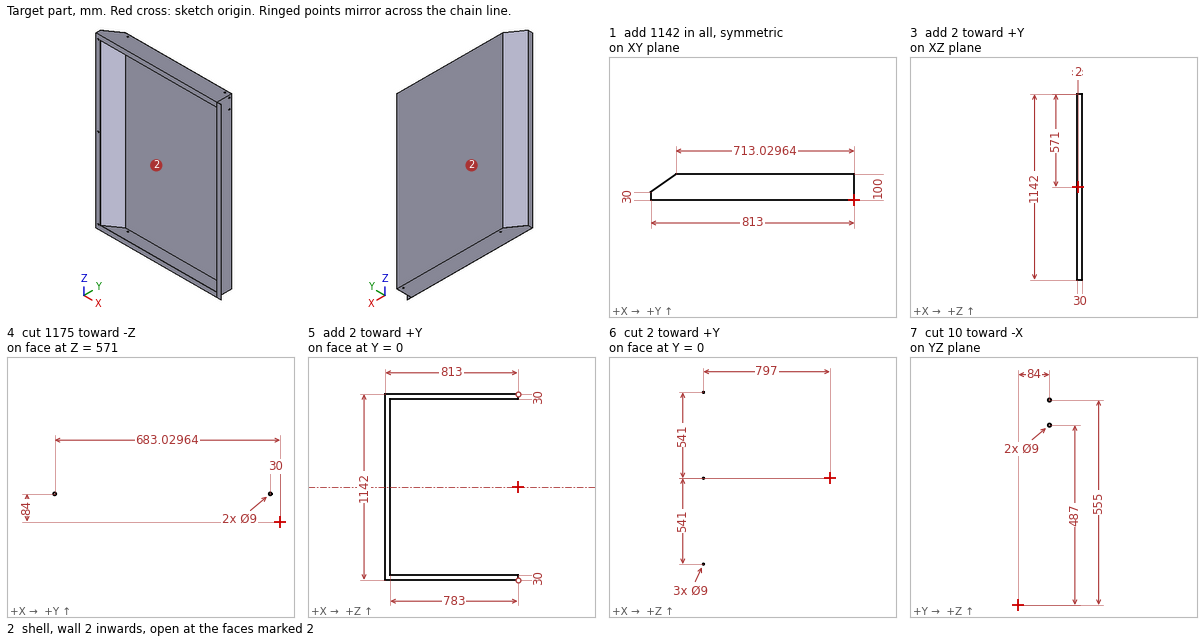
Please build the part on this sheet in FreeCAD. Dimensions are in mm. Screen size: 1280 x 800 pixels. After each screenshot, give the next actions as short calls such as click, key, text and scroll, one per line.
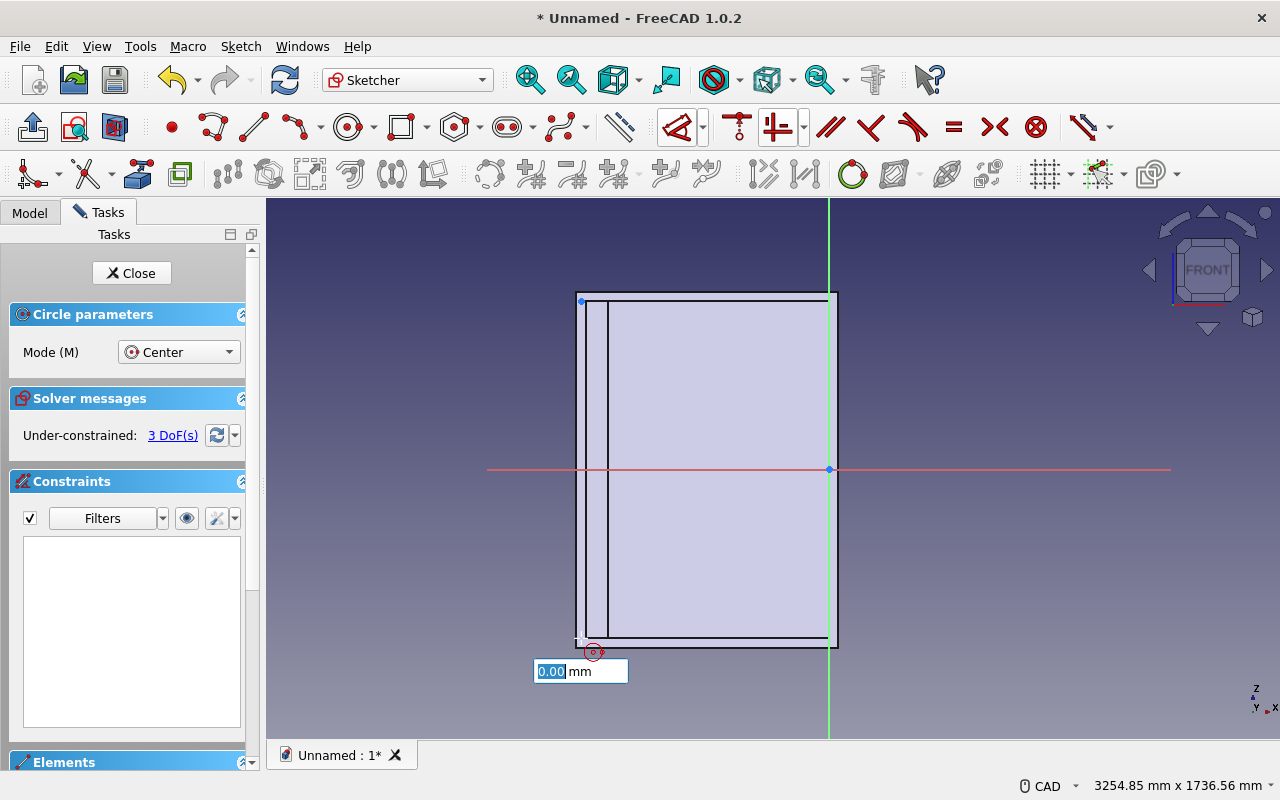
scroll(582, 637, up, 13)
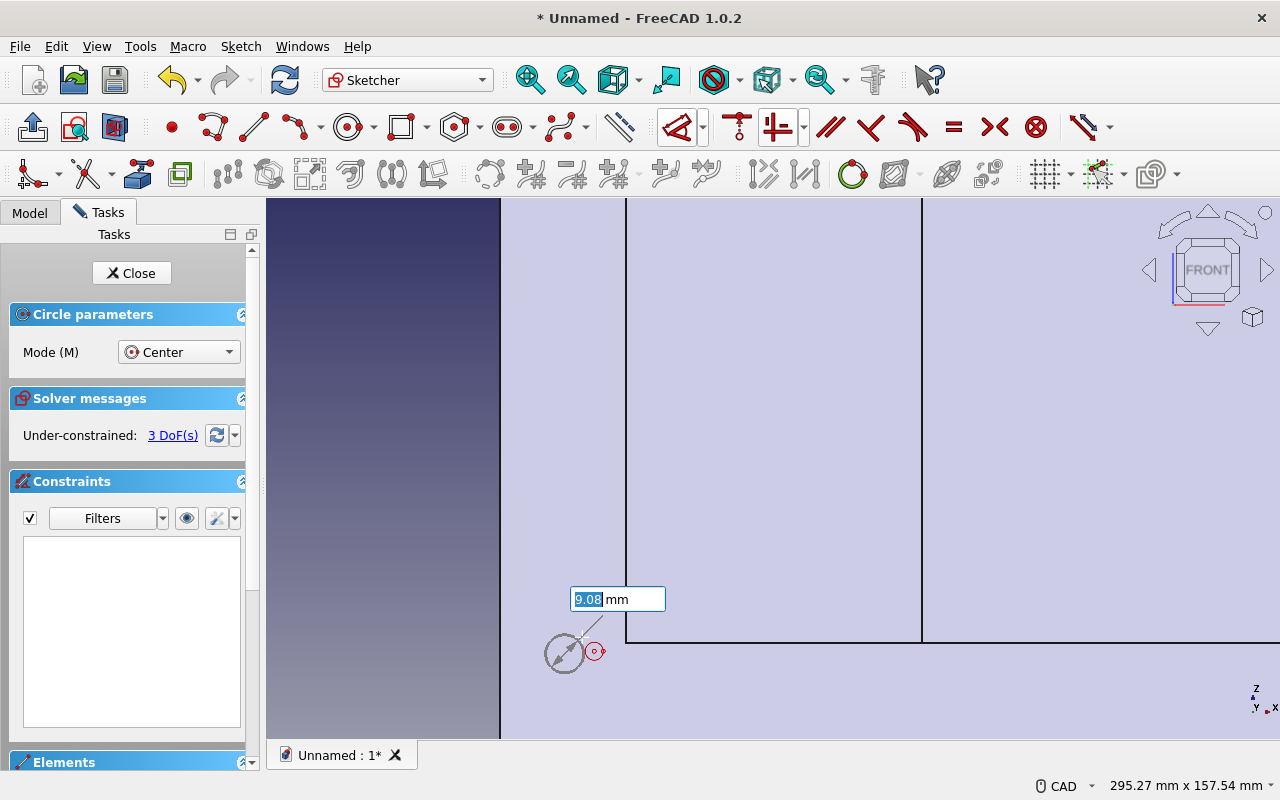
click(580, 629)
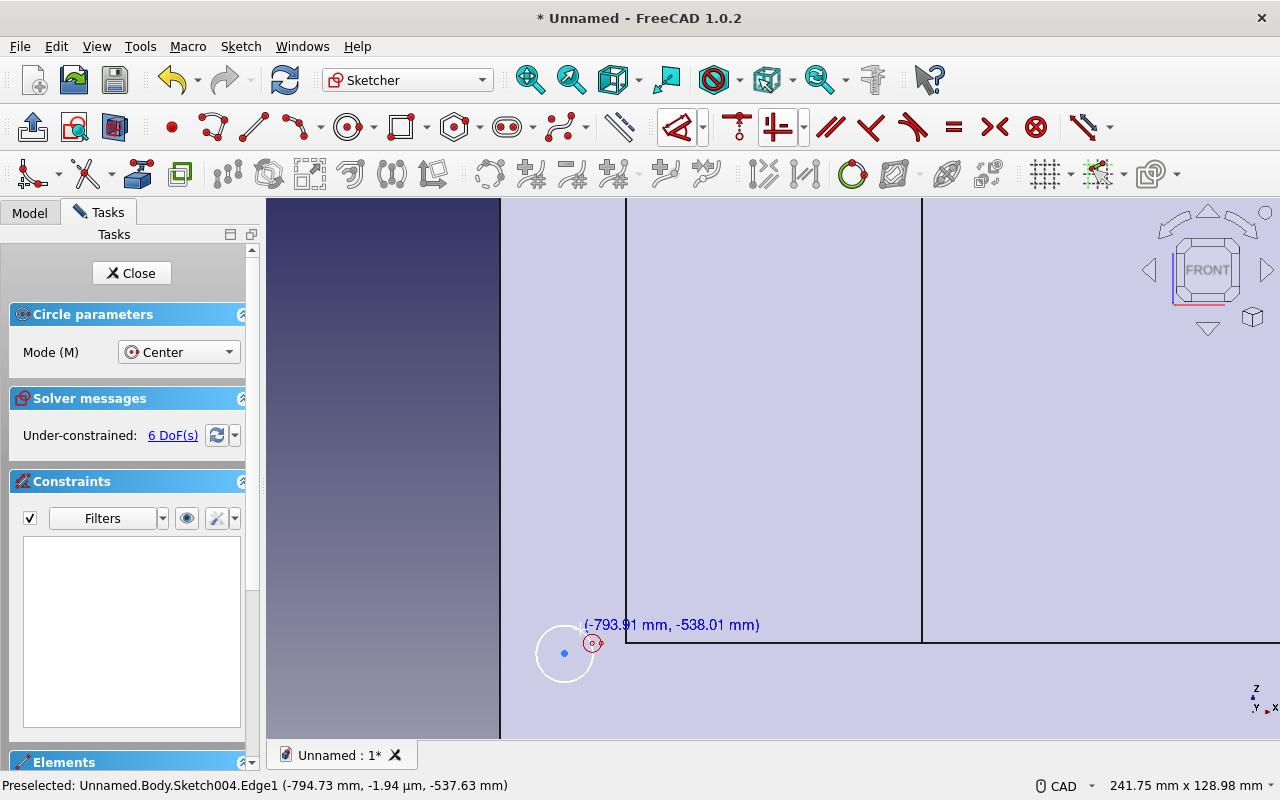
scroll(582, 637, down, 13)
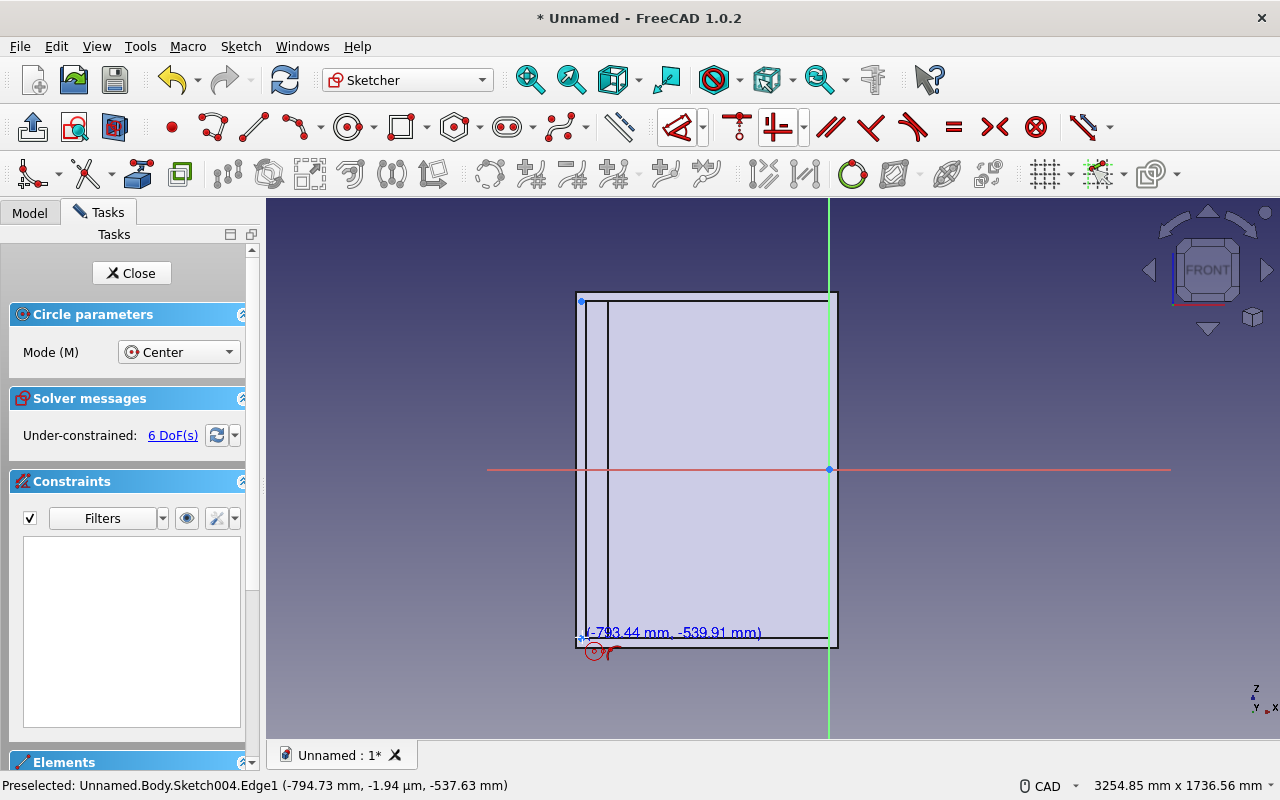
scroll(581, 470, up, 14)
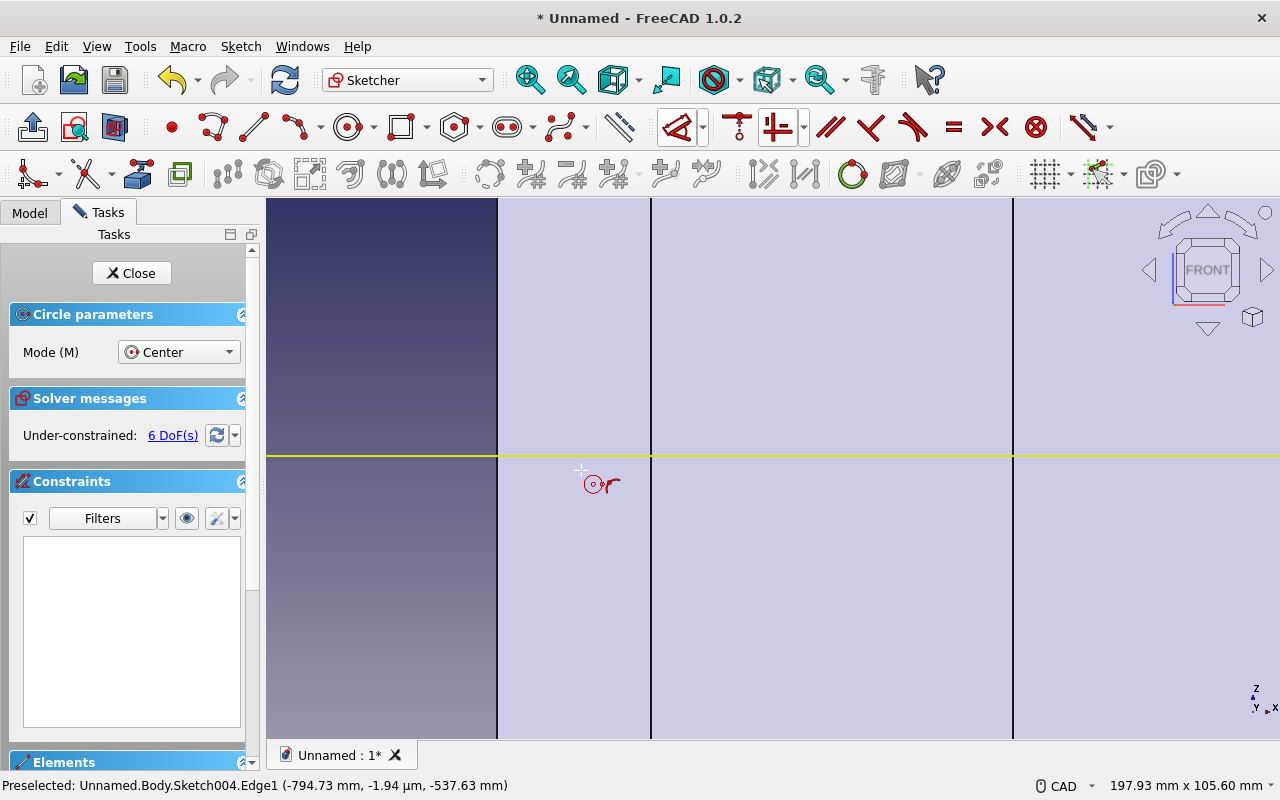
scroll(581, 469, down, 14)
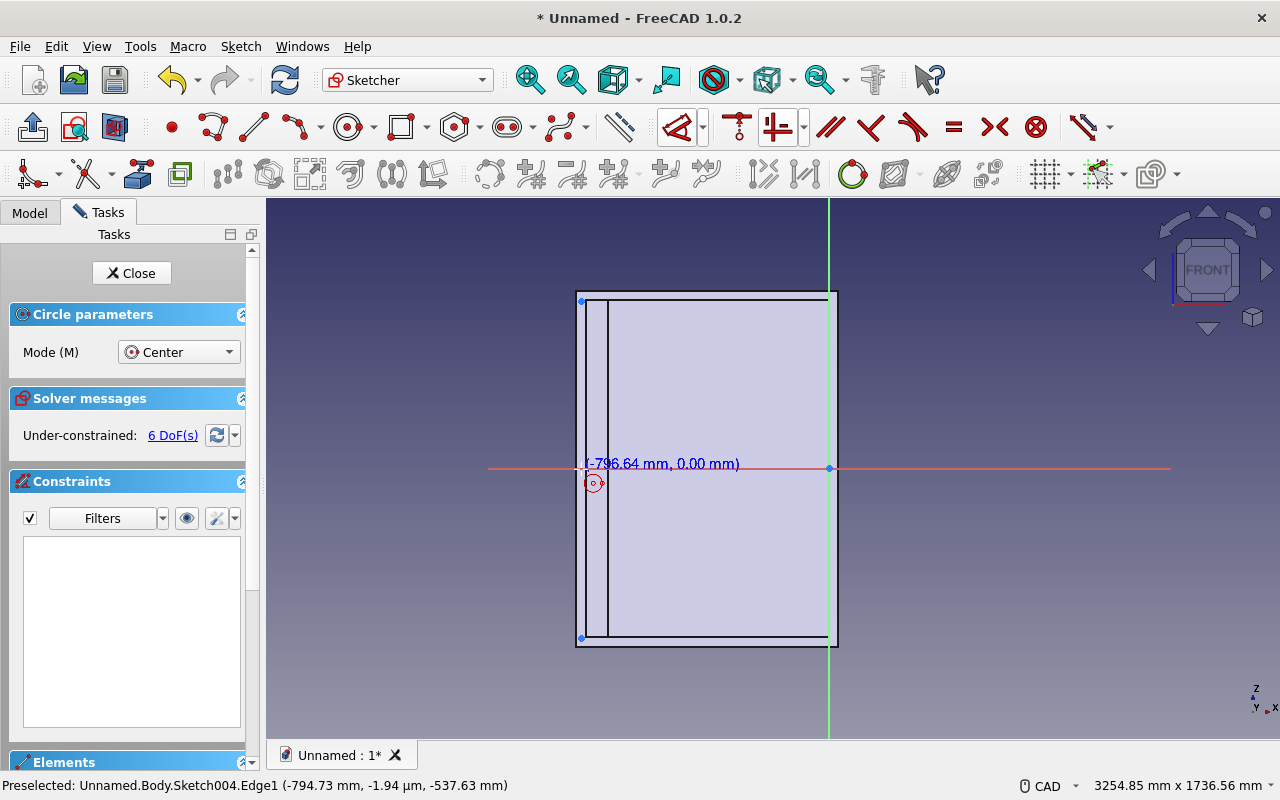
click(581, 469)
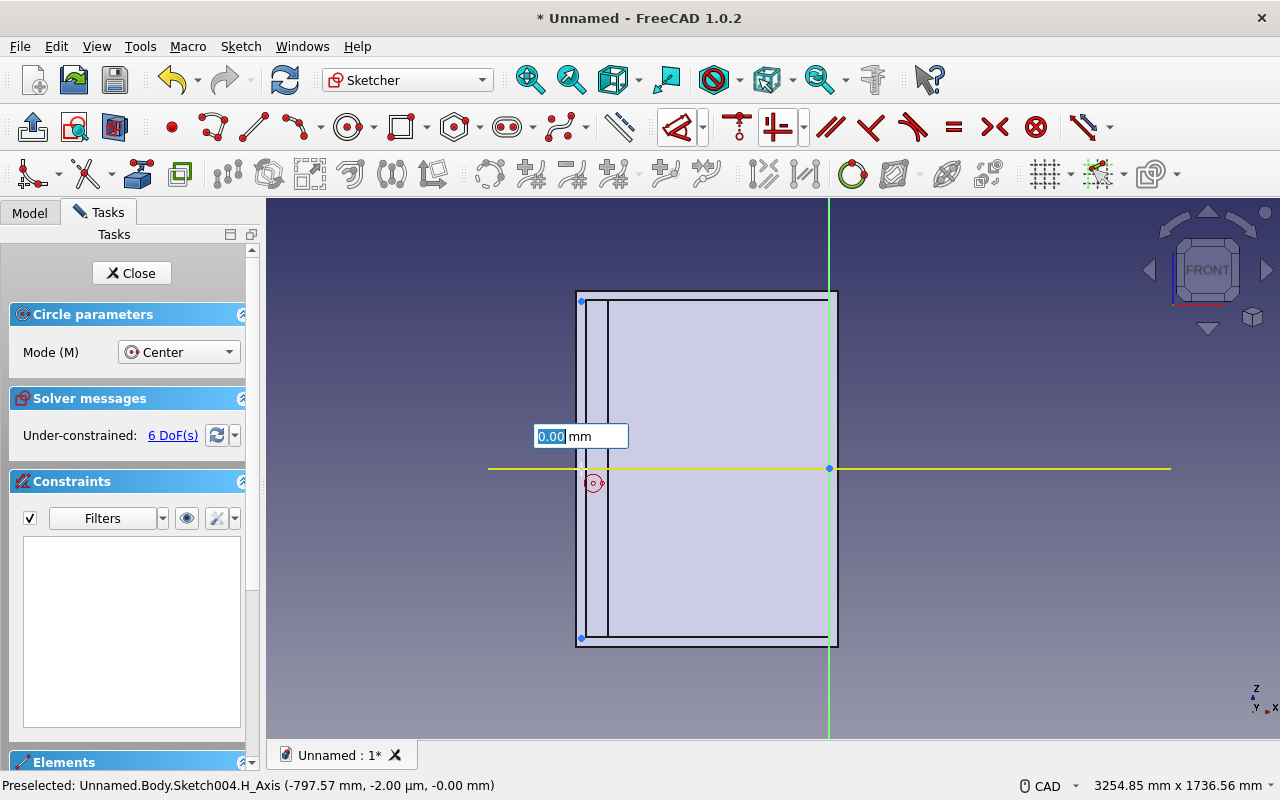
scroll(581, 470, up, 13)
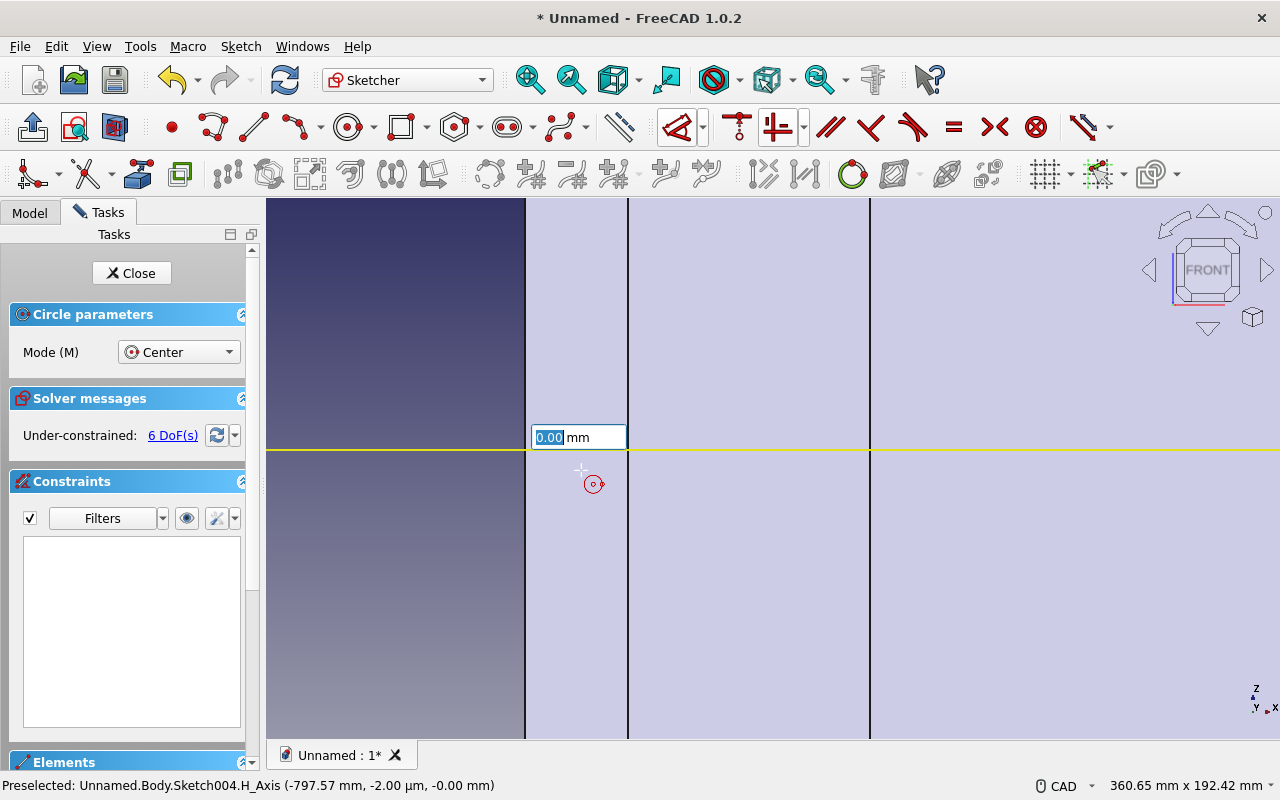
click(573, 464)
key(Escape)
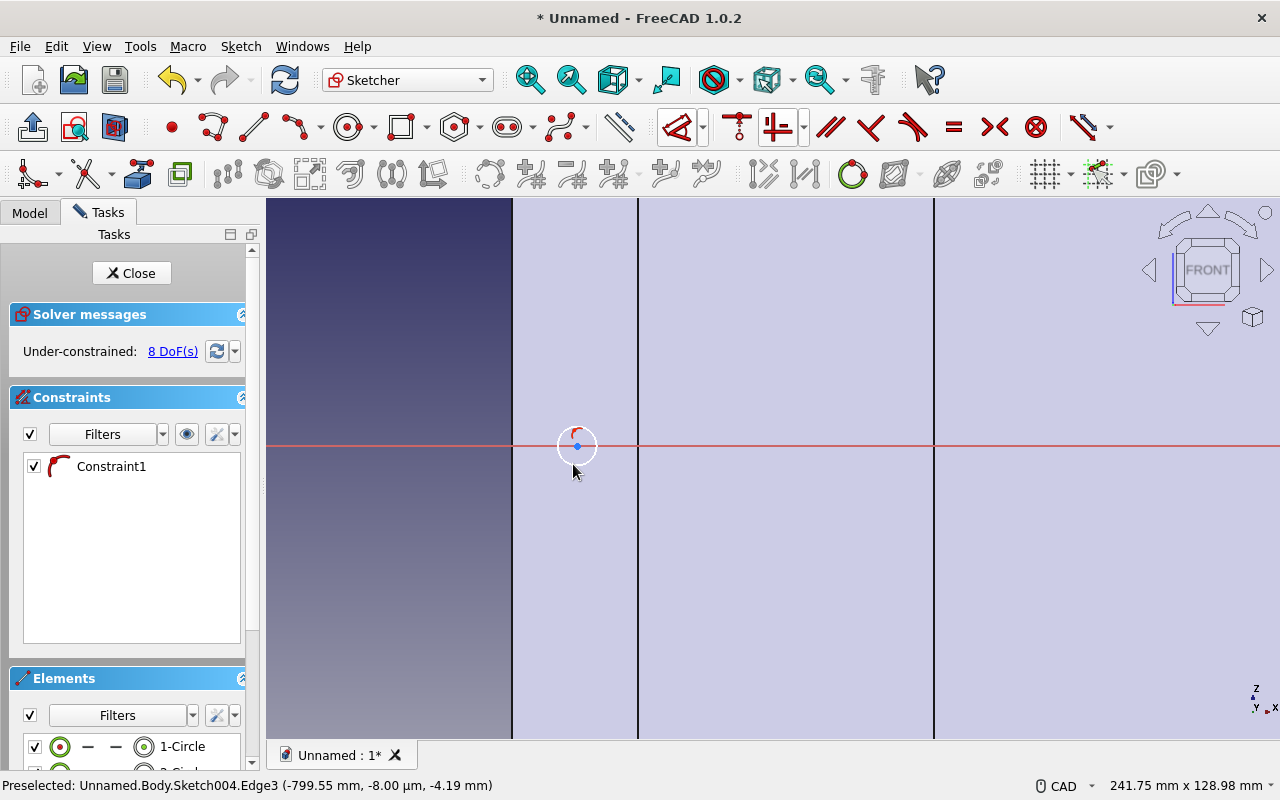
scroll(581, 470, down, 13)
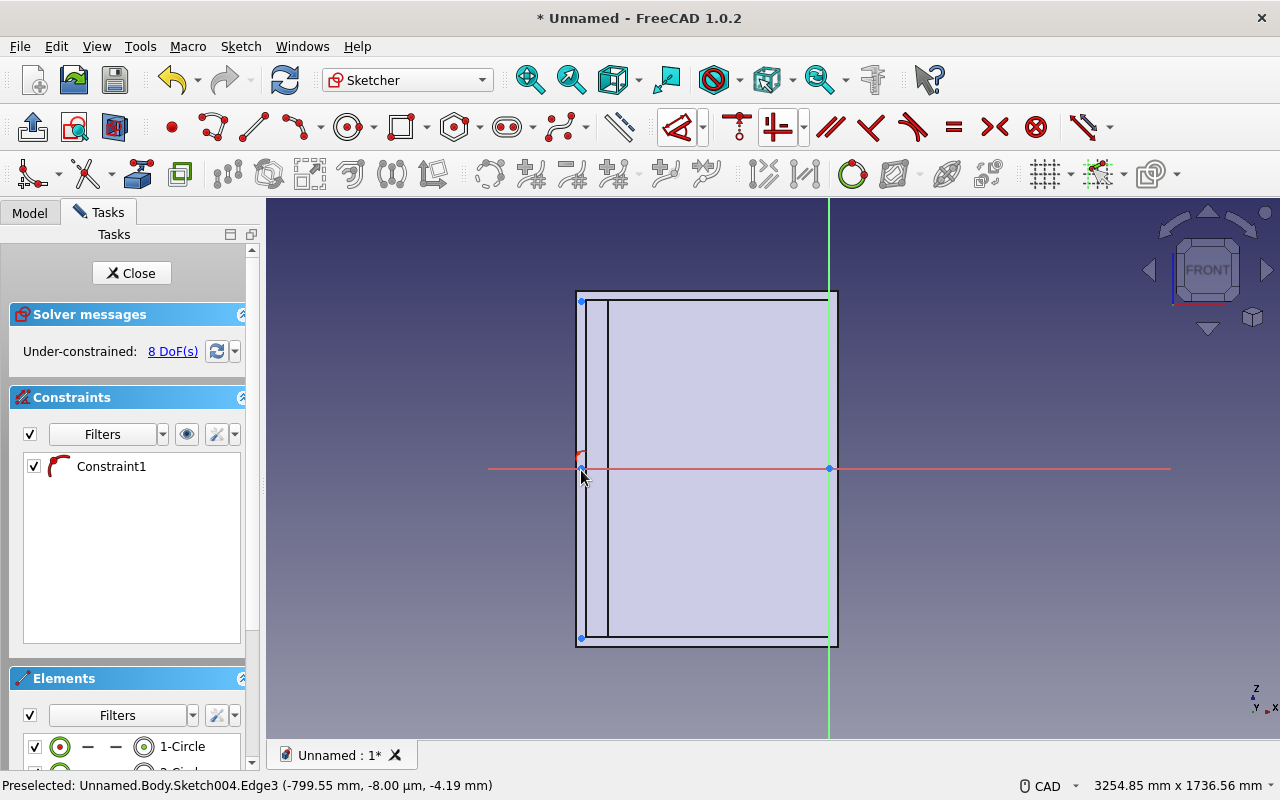
scroll(582, 300, up, 10)